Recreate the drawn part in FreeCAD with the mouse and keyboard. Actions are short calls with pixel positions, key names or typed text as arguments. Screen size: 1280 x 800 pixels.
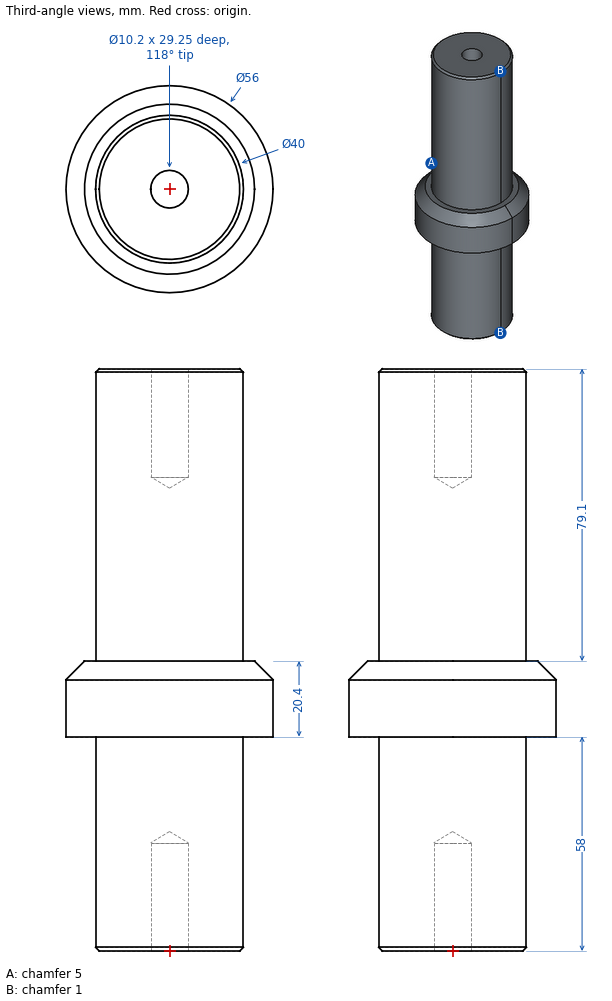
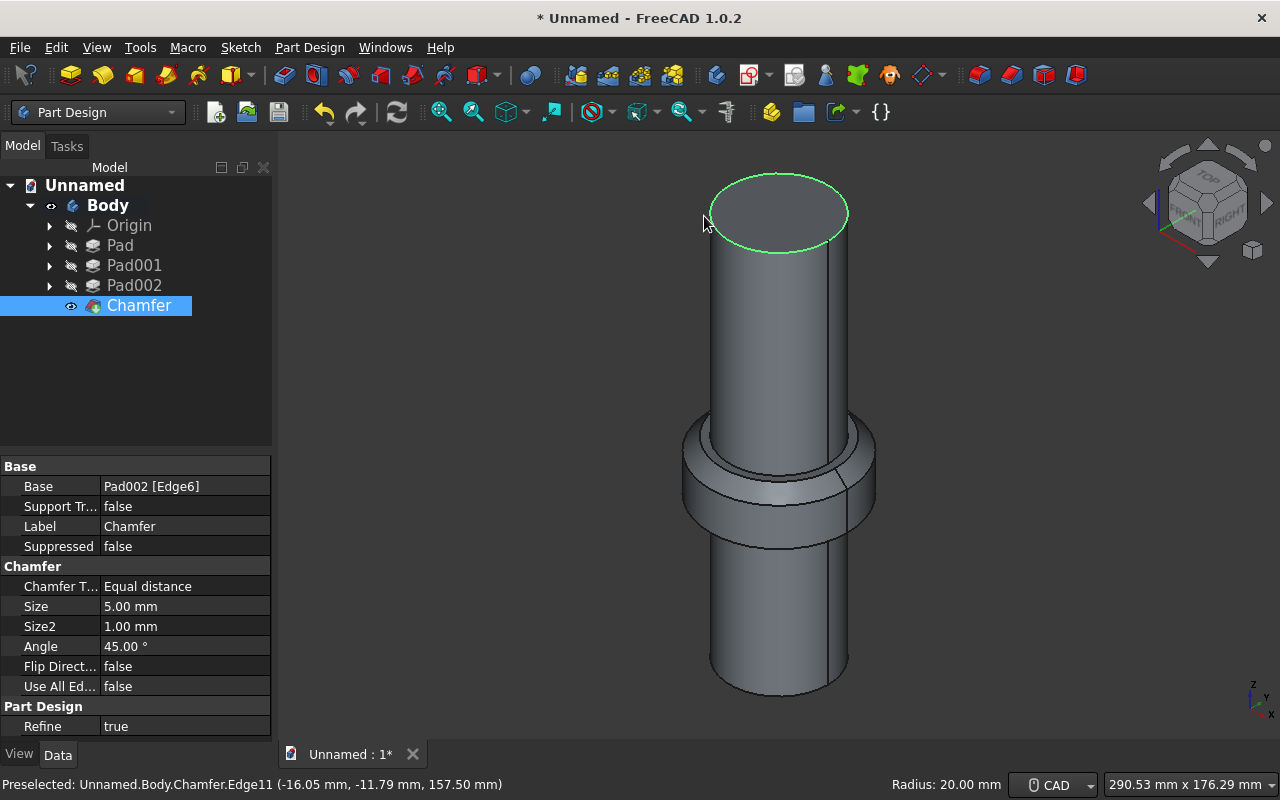
key(2)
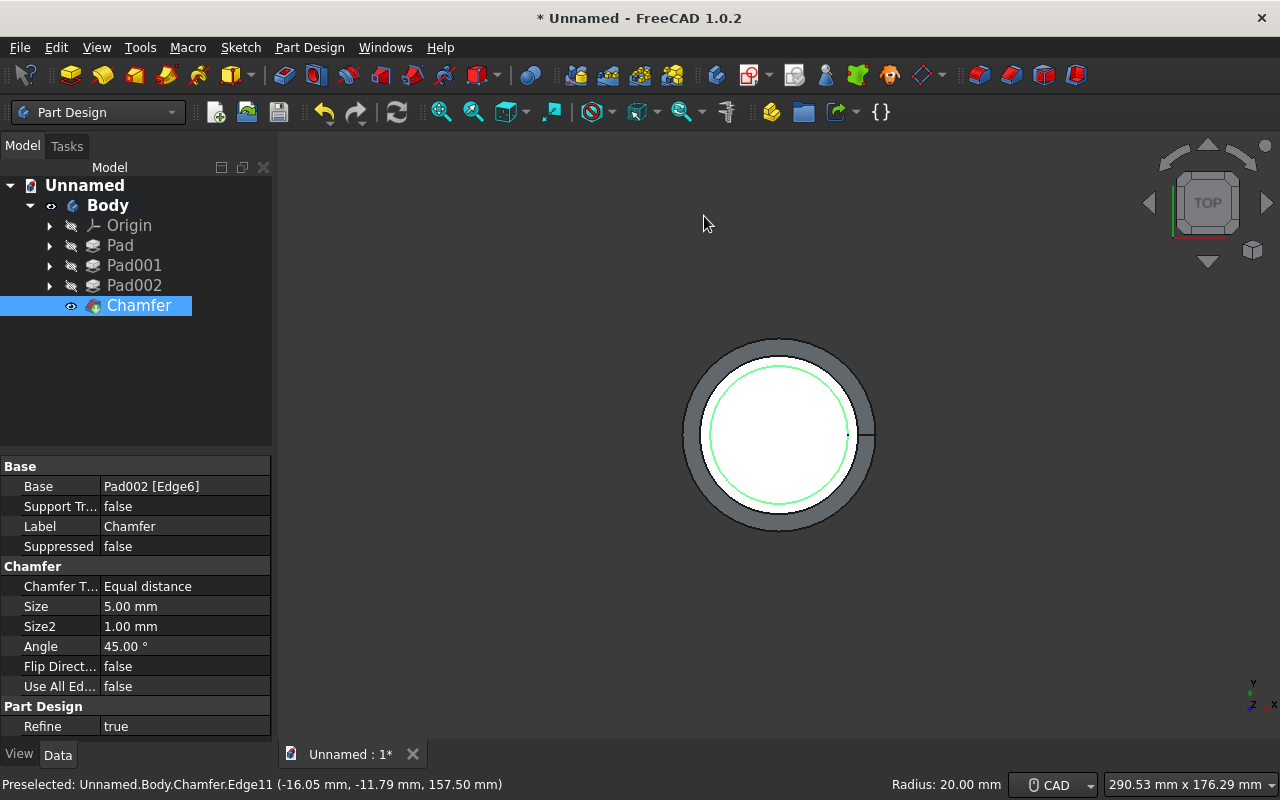
click(442, 112)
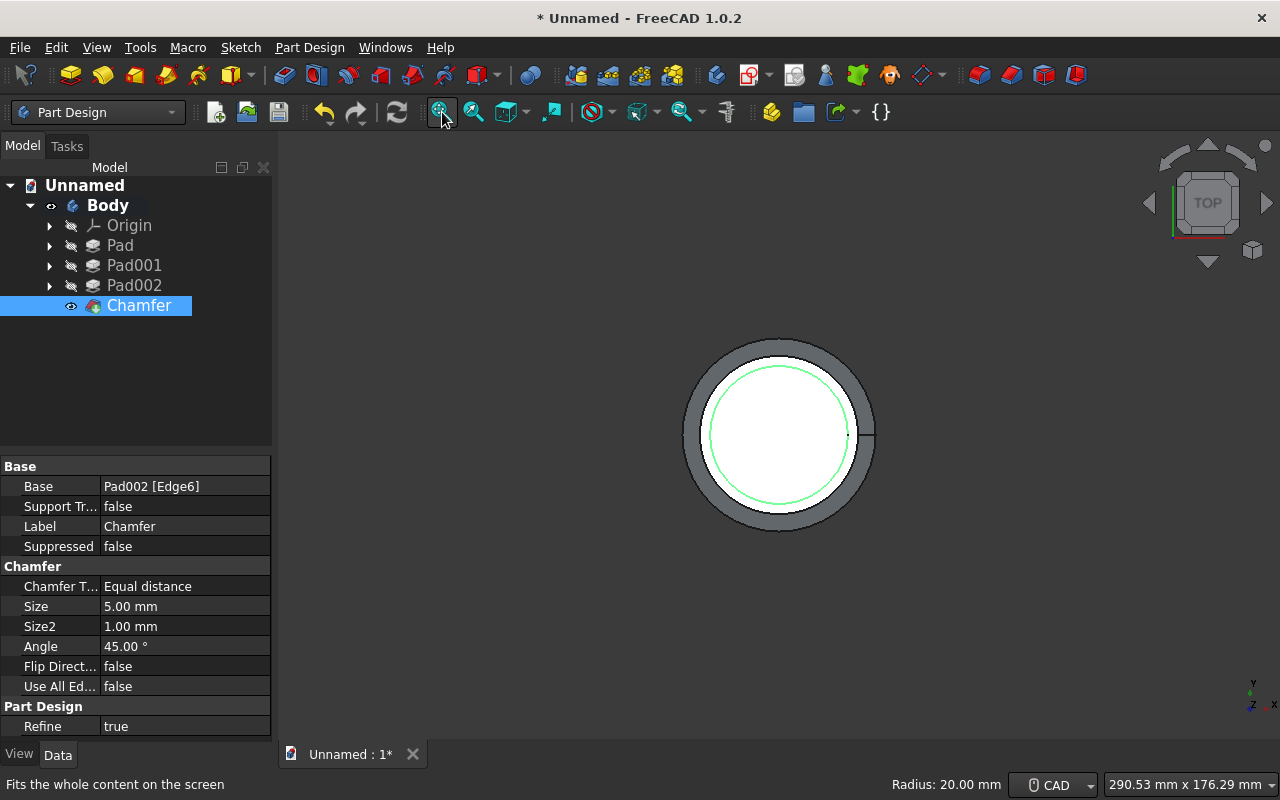
key(1)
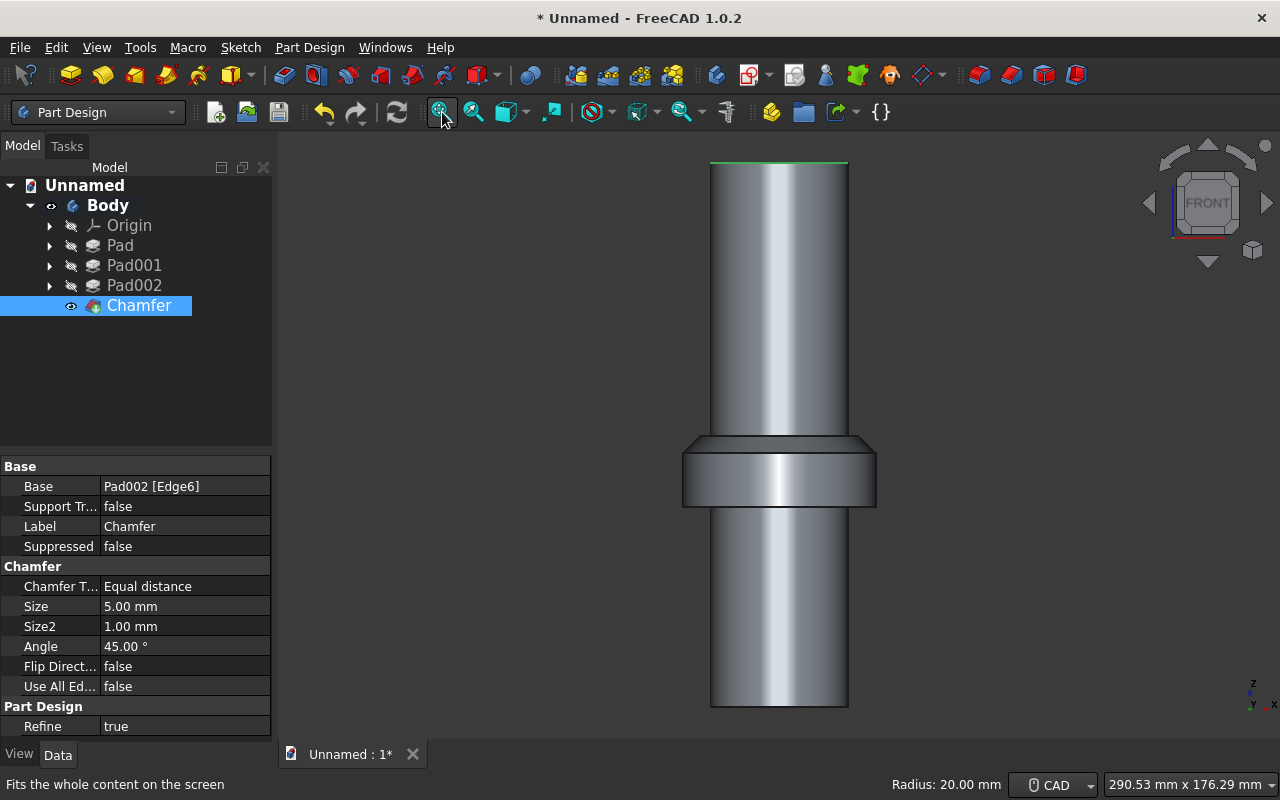
click(723, 706, ctrl)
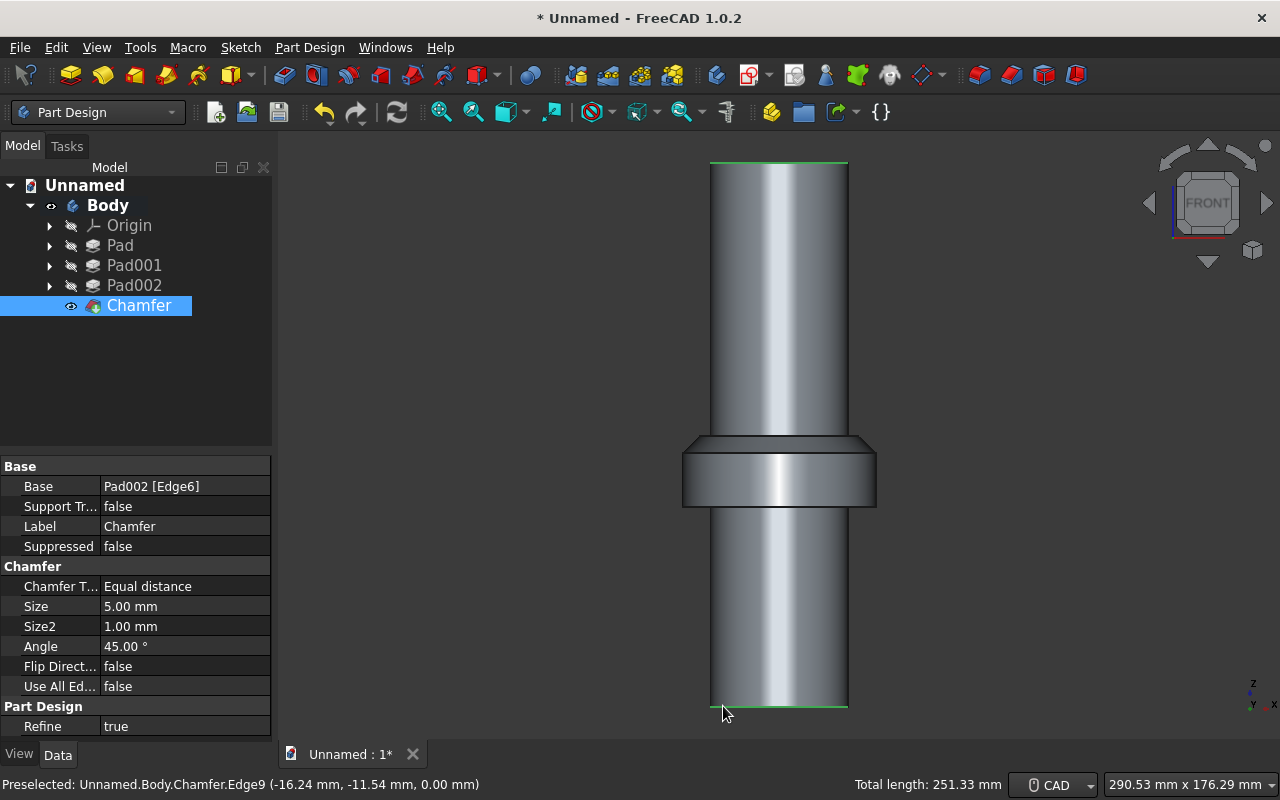
click(1012, 76)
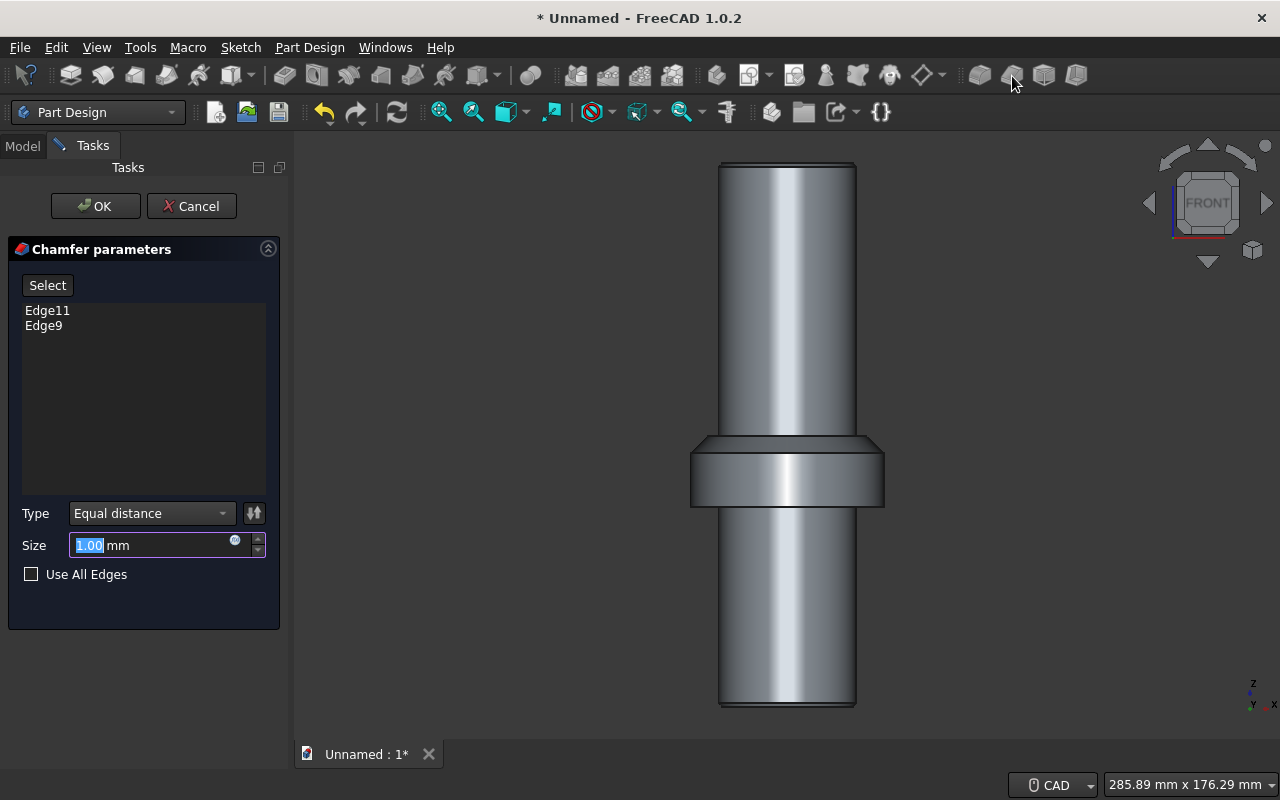
text(1)
key(Tab)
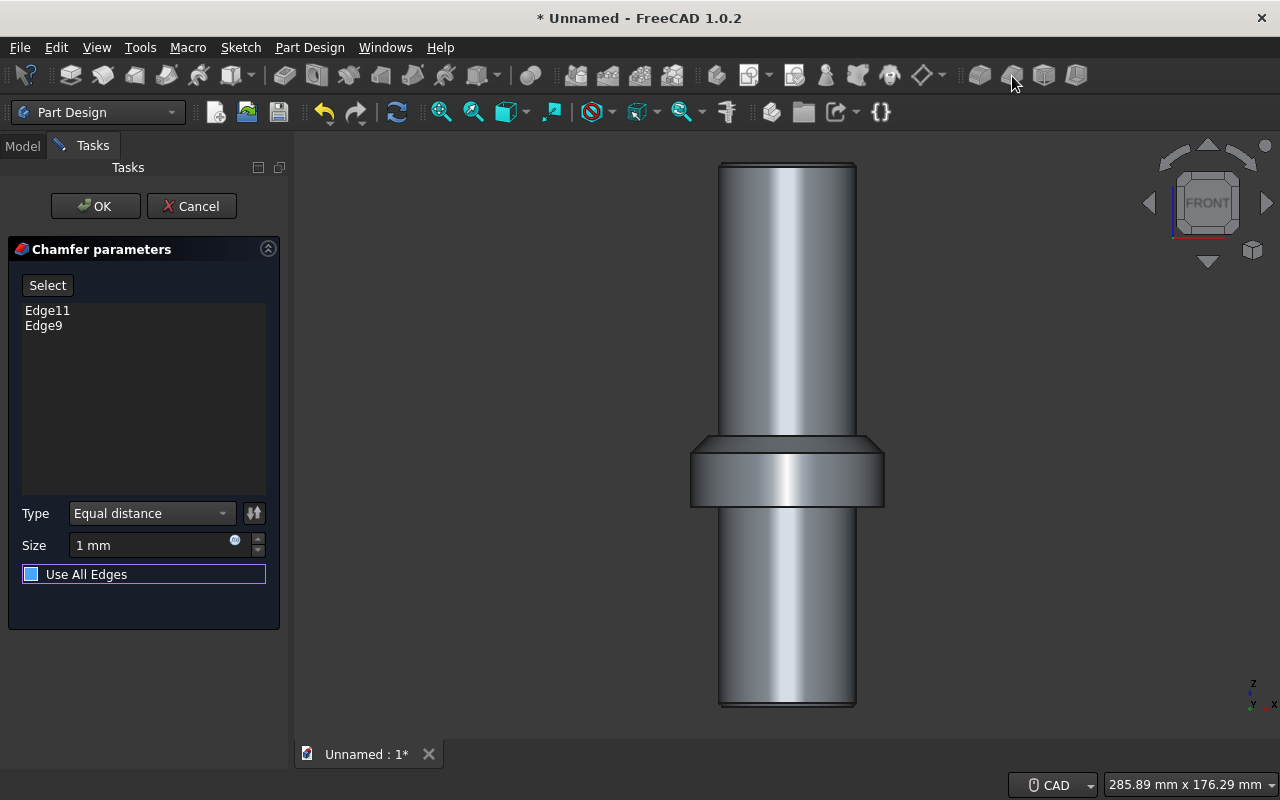
click(96, 206)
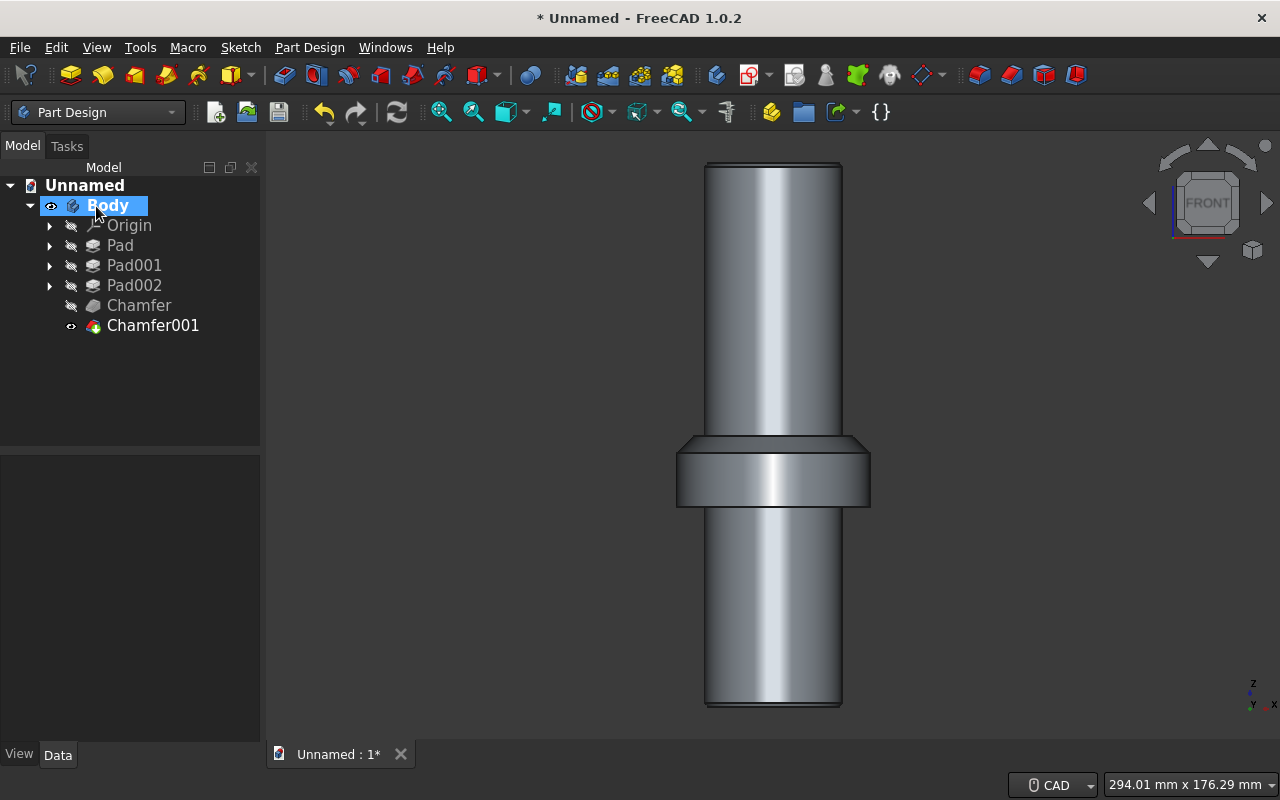
key(5)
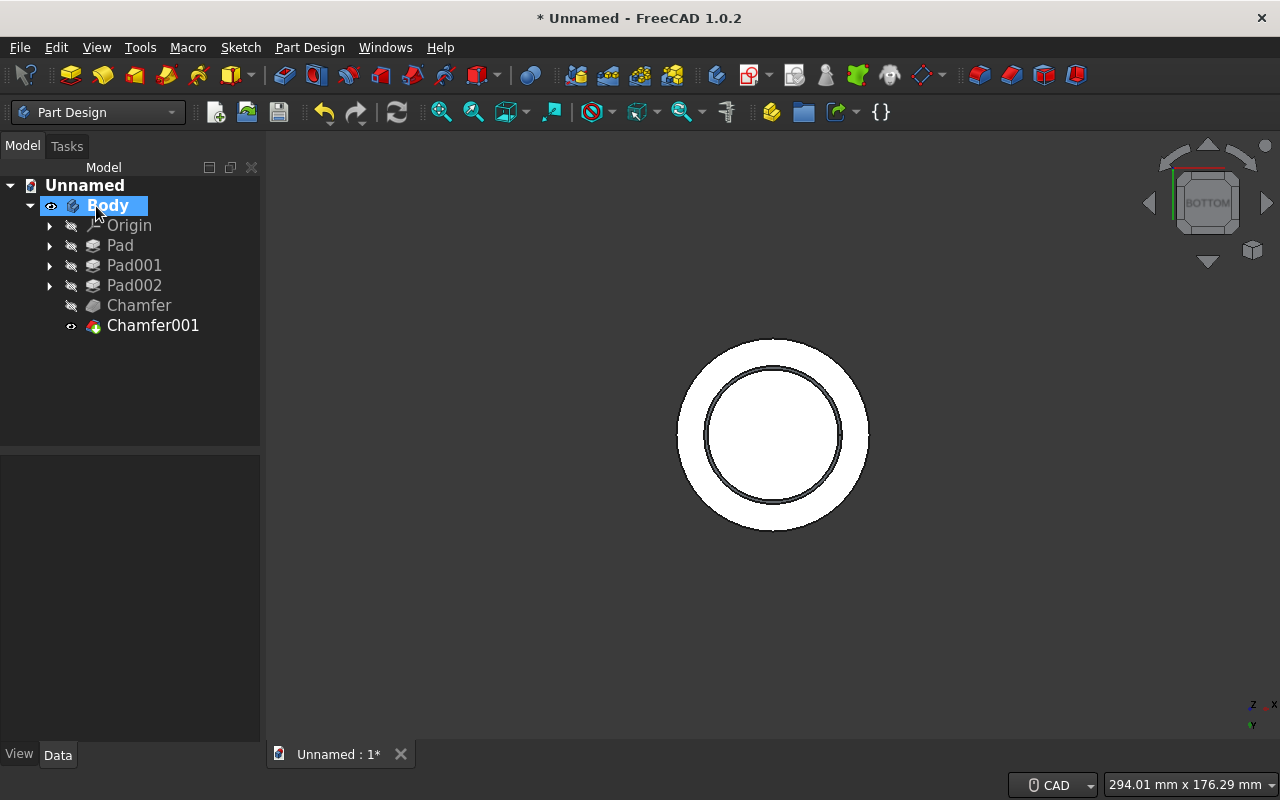
click(442, 112)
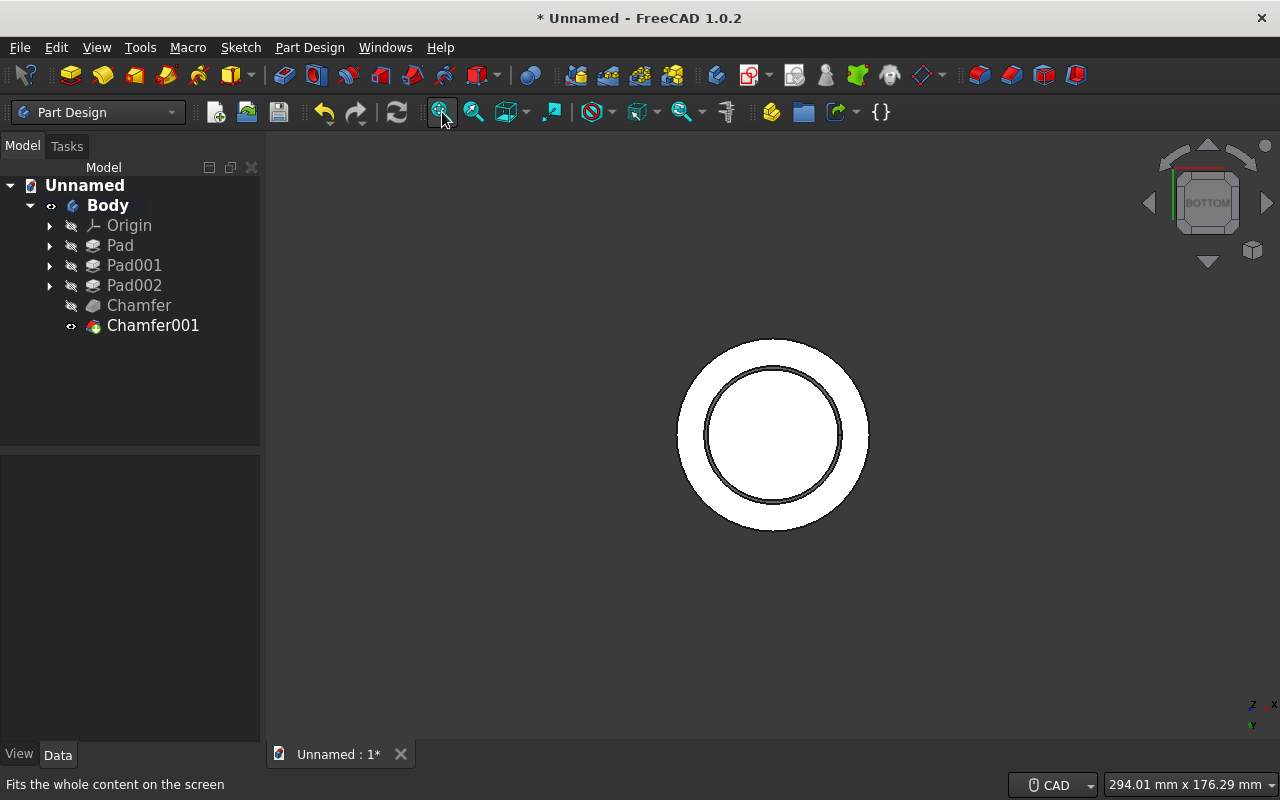
click(773, 434)